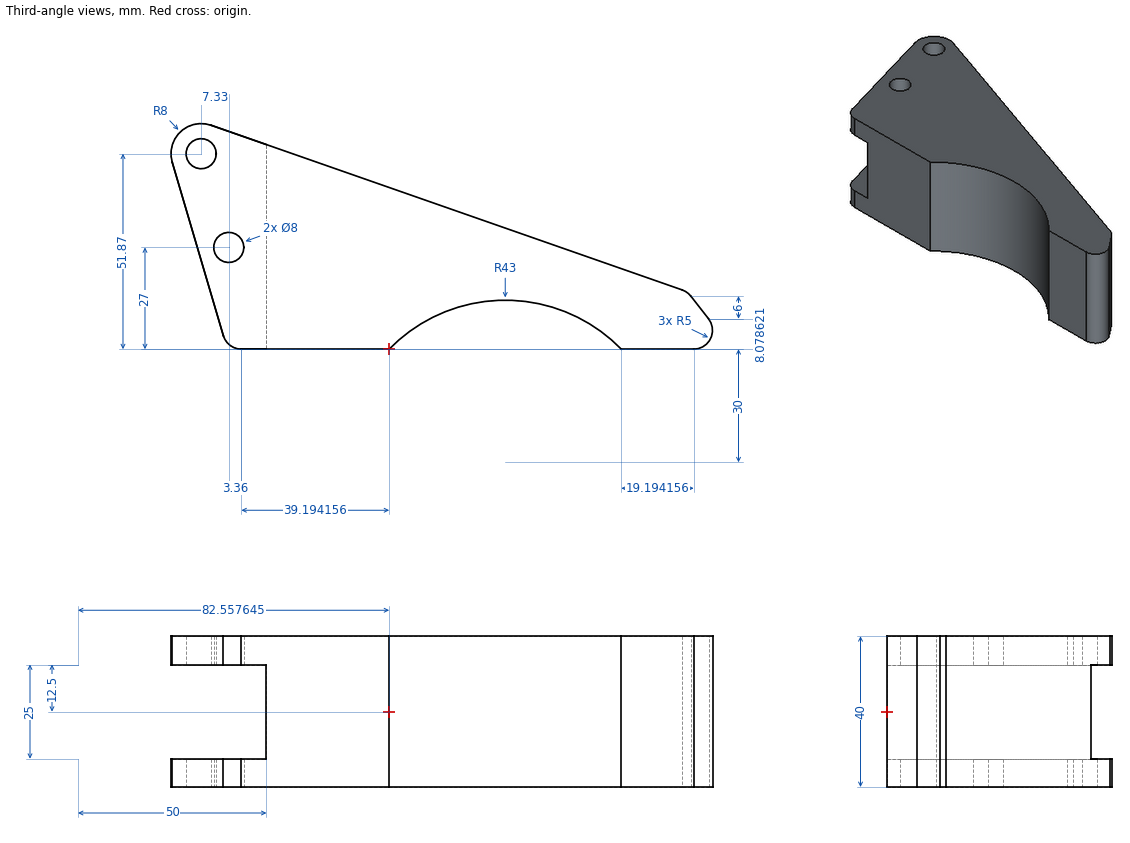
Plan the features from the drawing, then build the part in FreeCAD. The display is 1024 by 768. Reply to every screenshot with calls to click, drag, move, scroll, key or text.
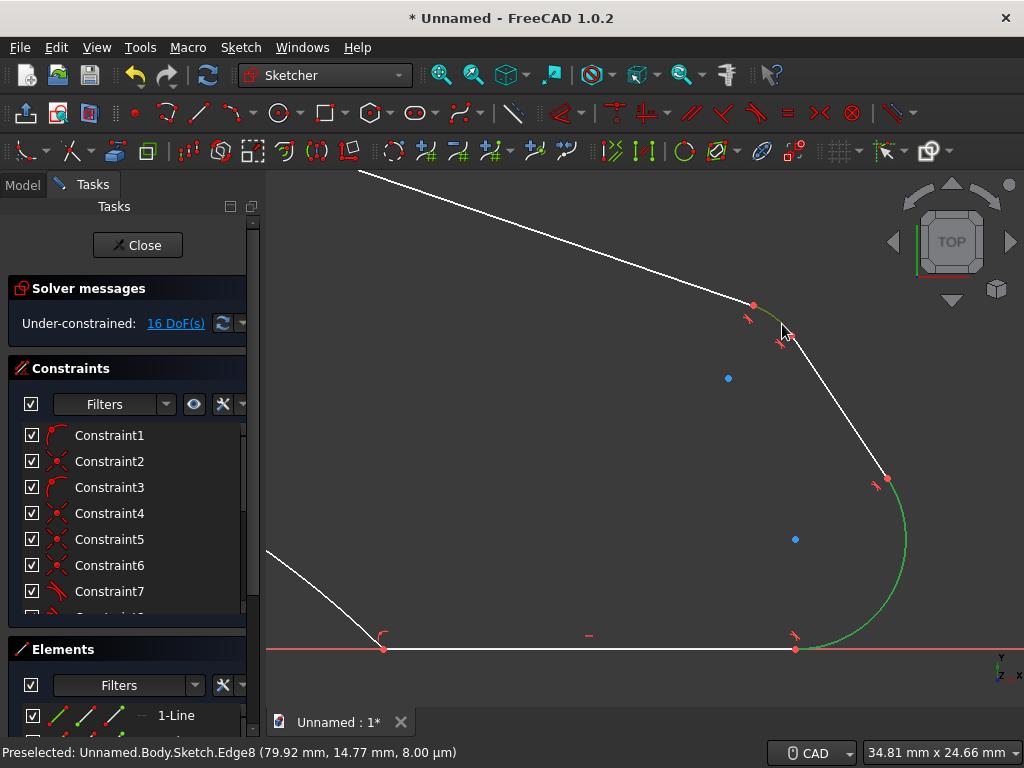
scroll(769, 507, down, 10)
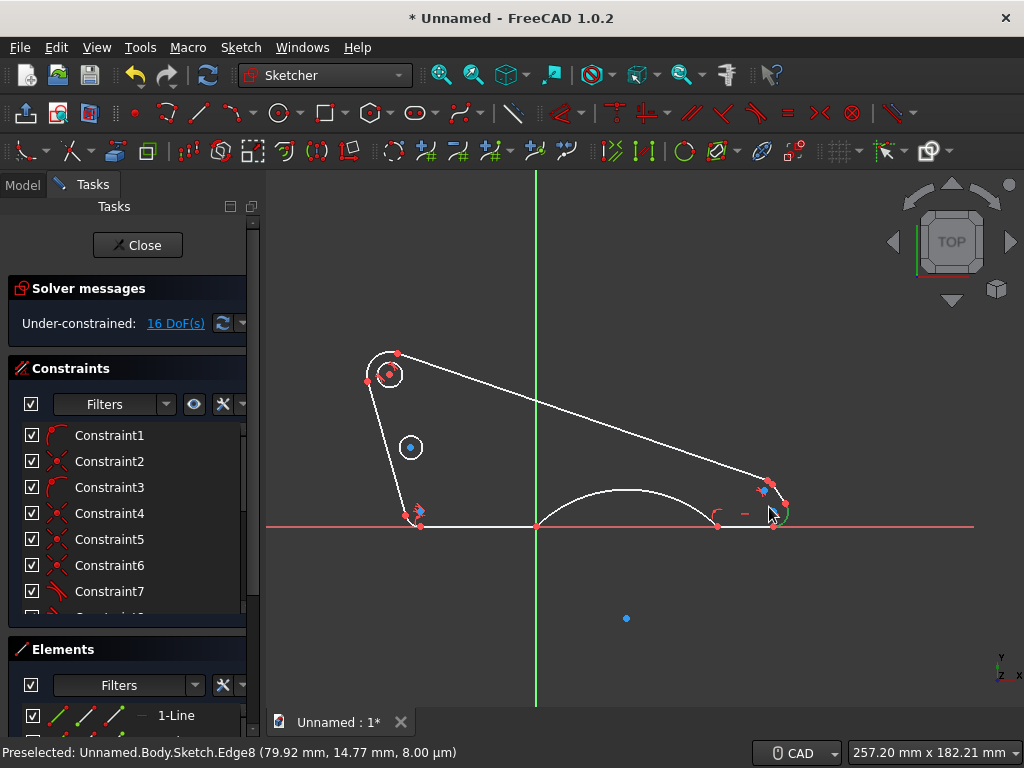
scroll(409, 521, up, 5)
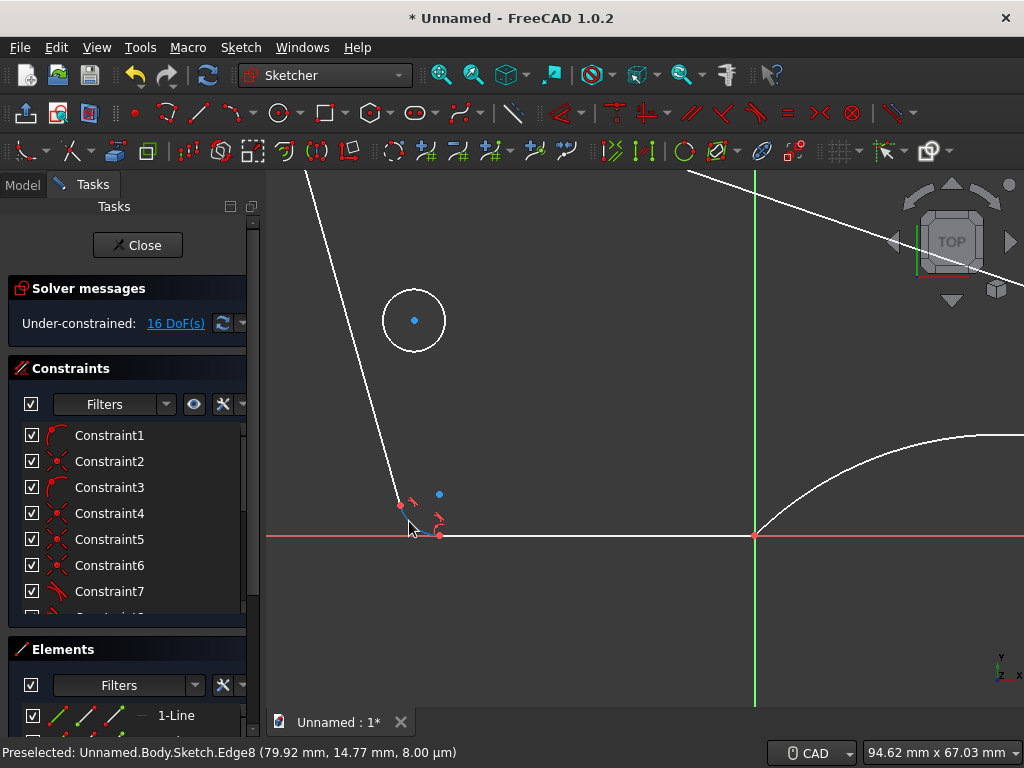
click(408, 520)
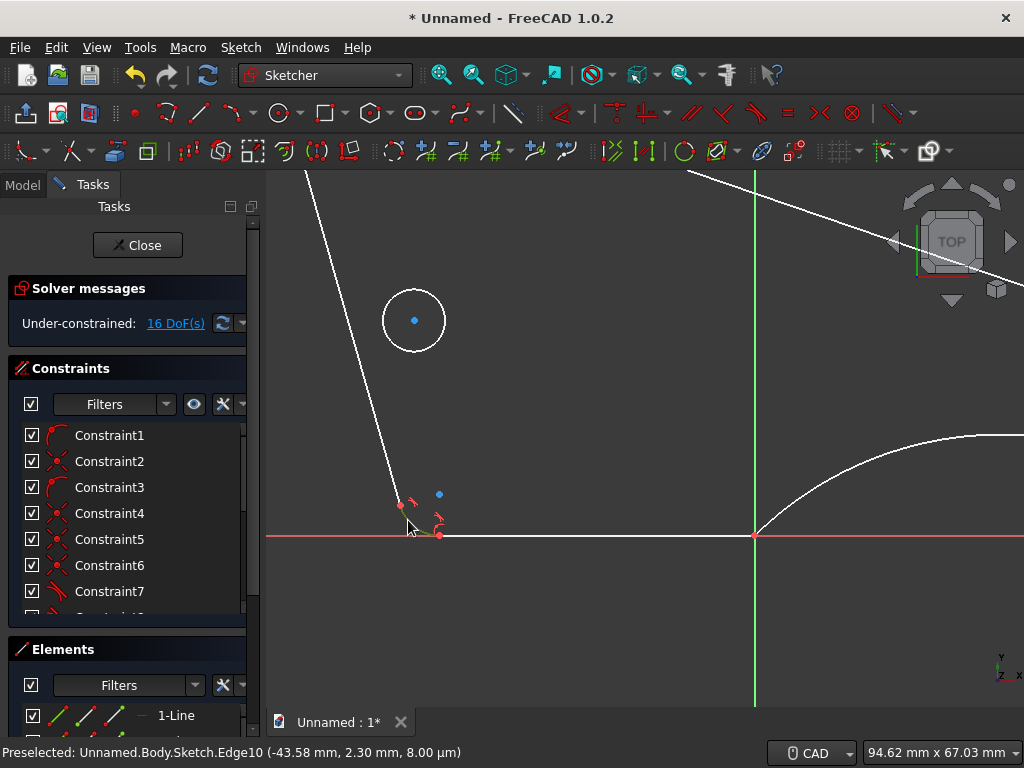
key(e)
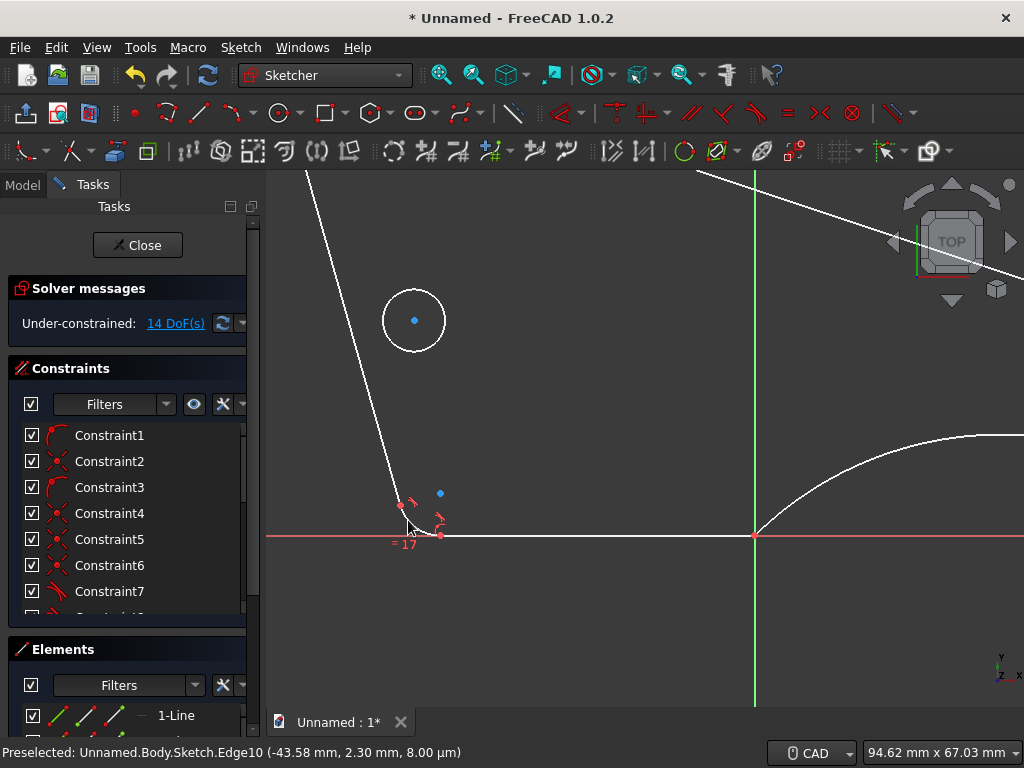
click(436, 298)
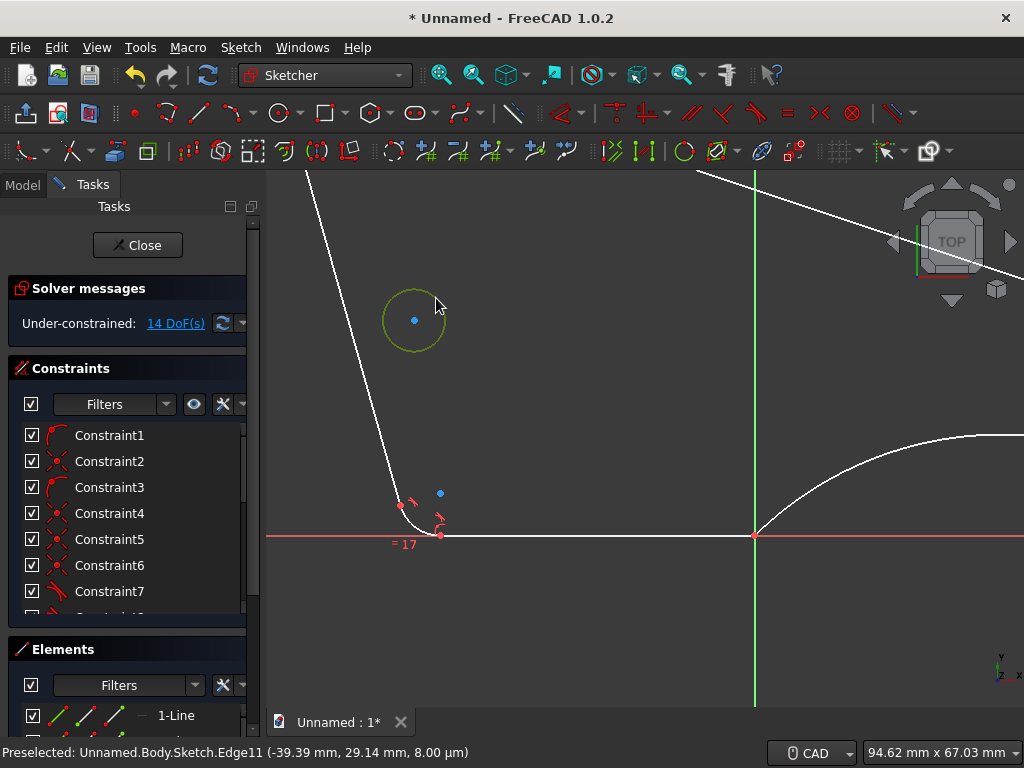
scroll(408, 520, down, 5)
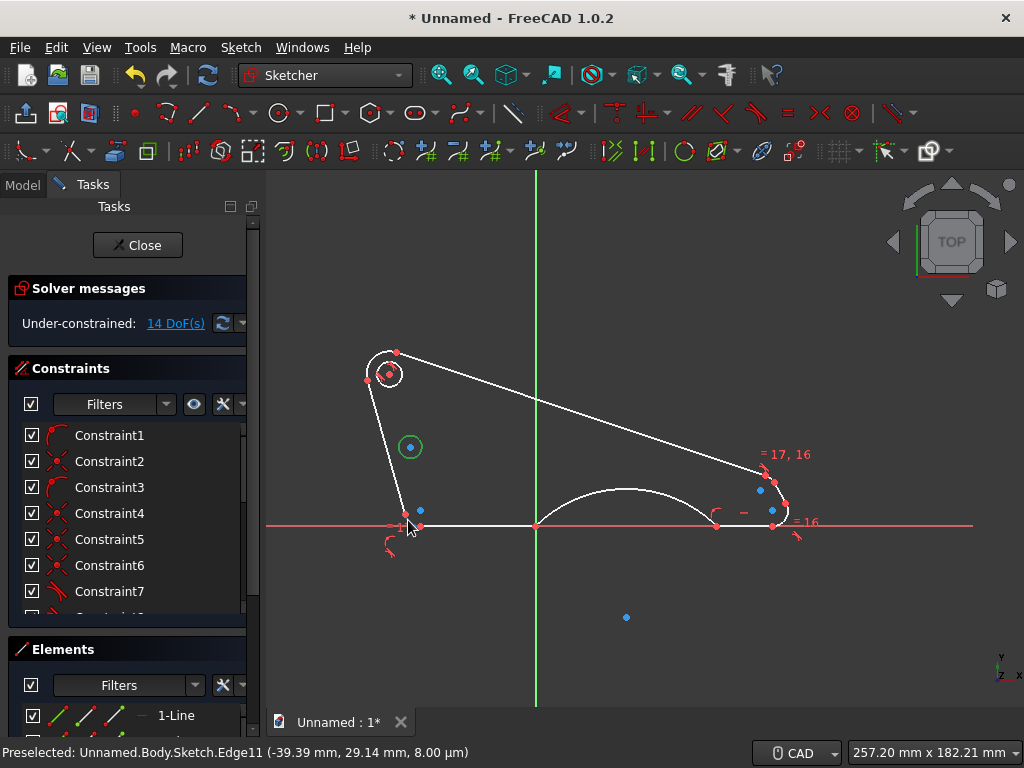
click(381, 366)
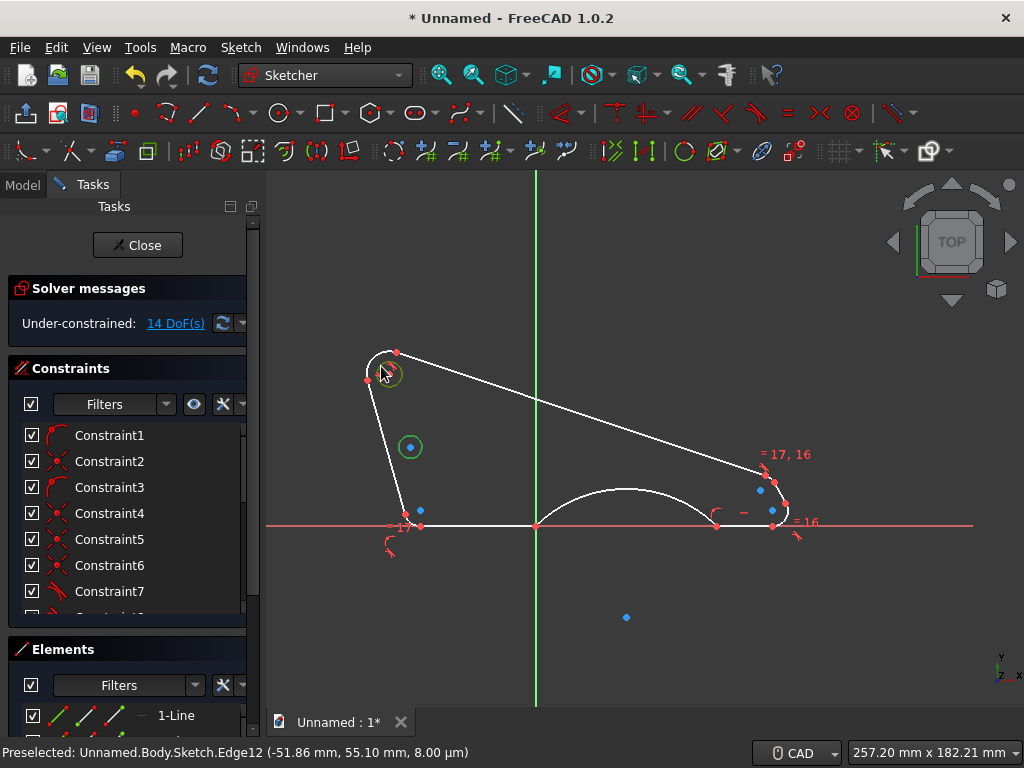
click(788, 114)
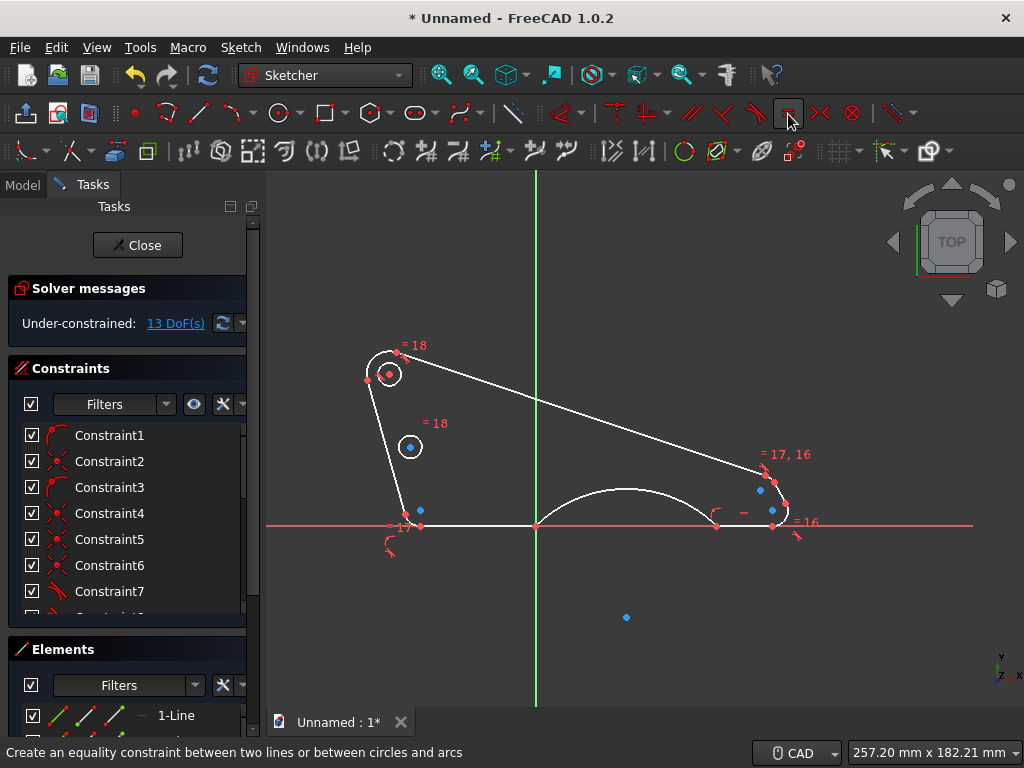
click(666, 495)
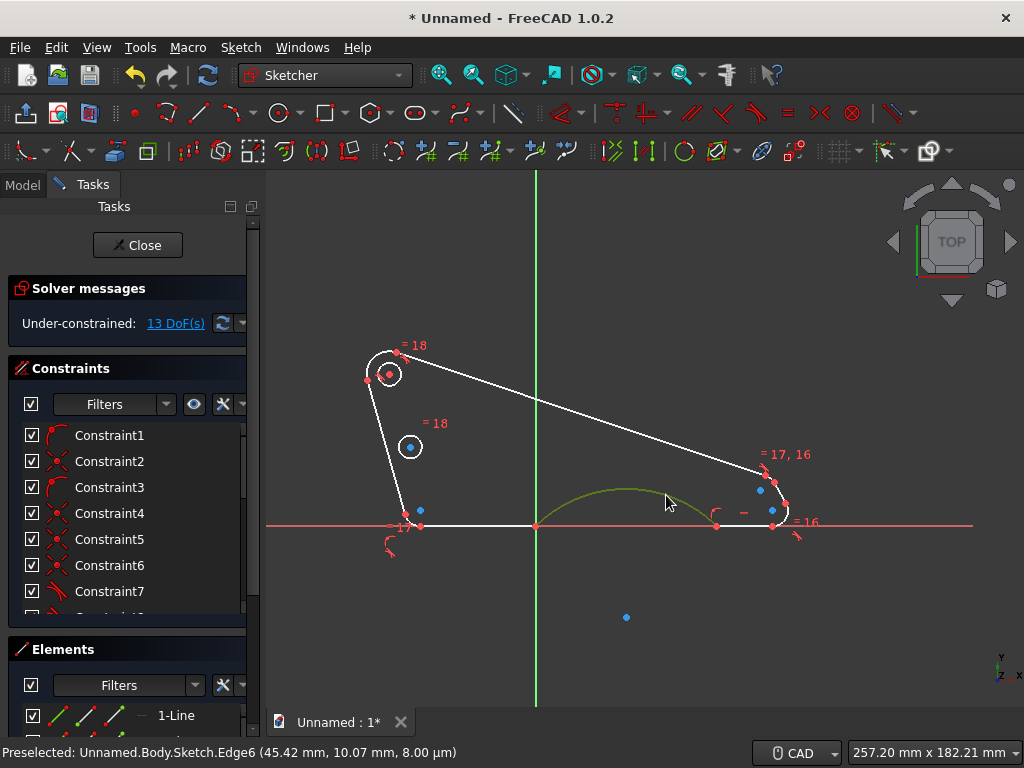
click(584, 114)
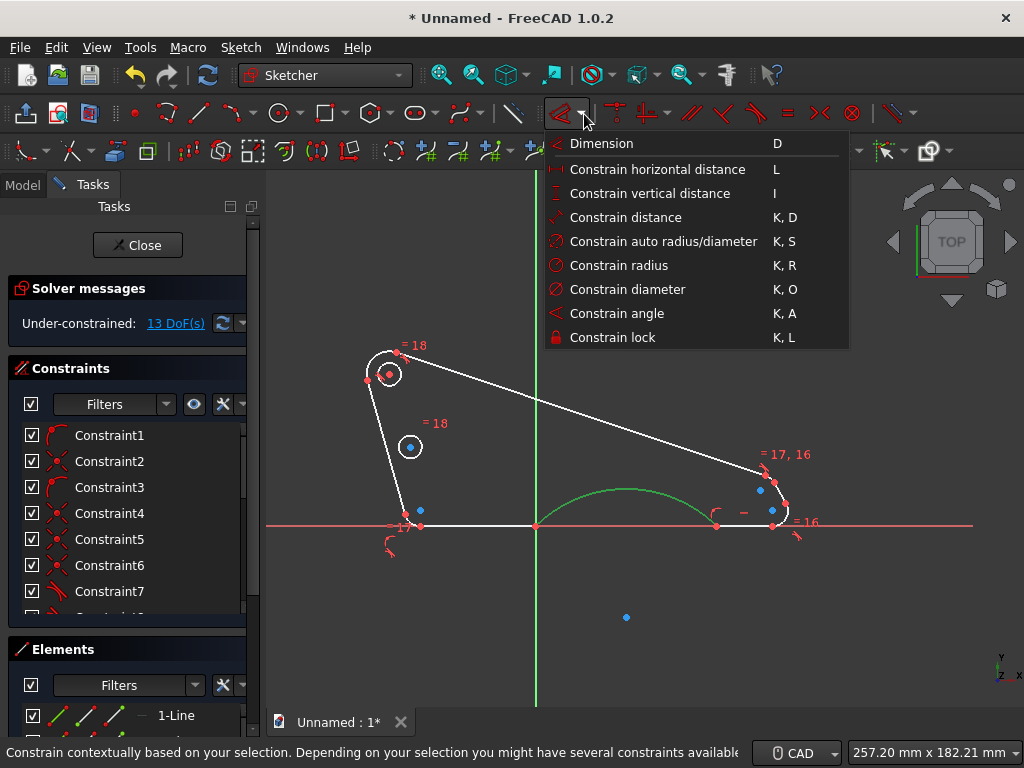
click(697, 265)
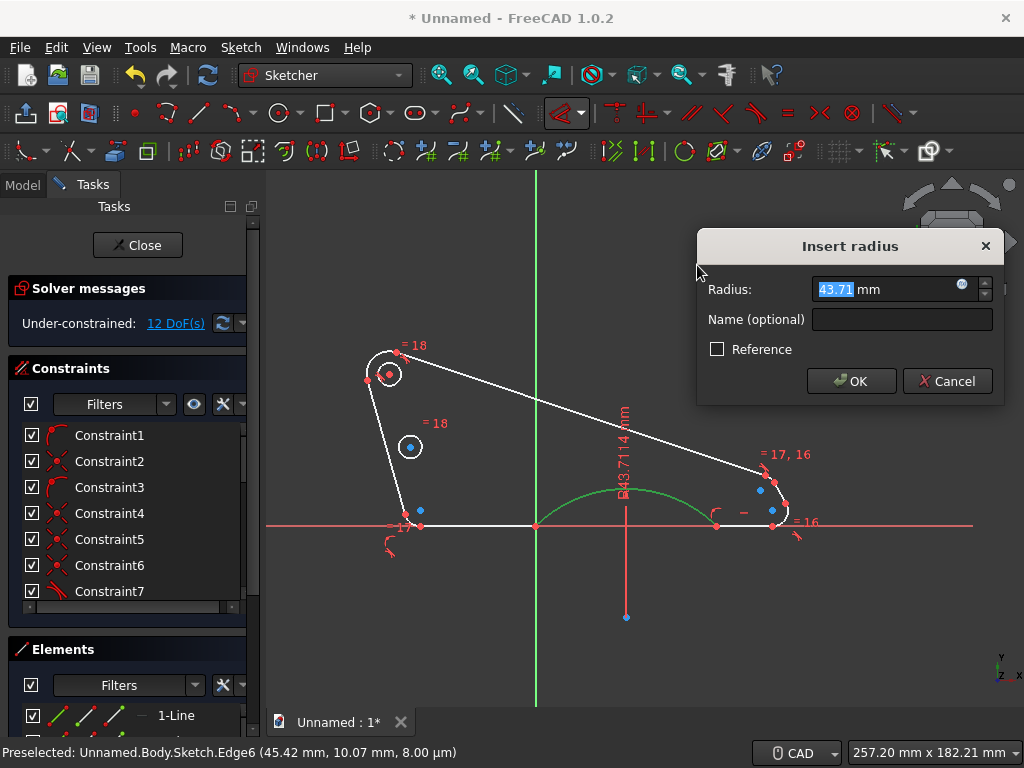
text(43)
key(Return)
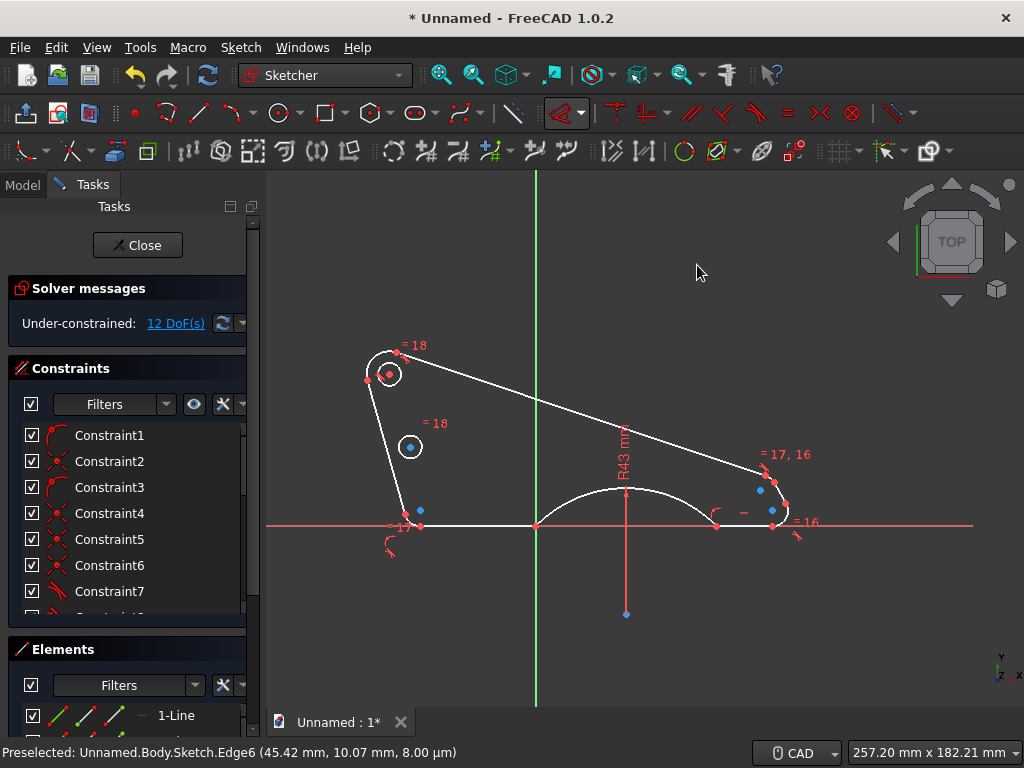
scroll(782, 523, up, 5)